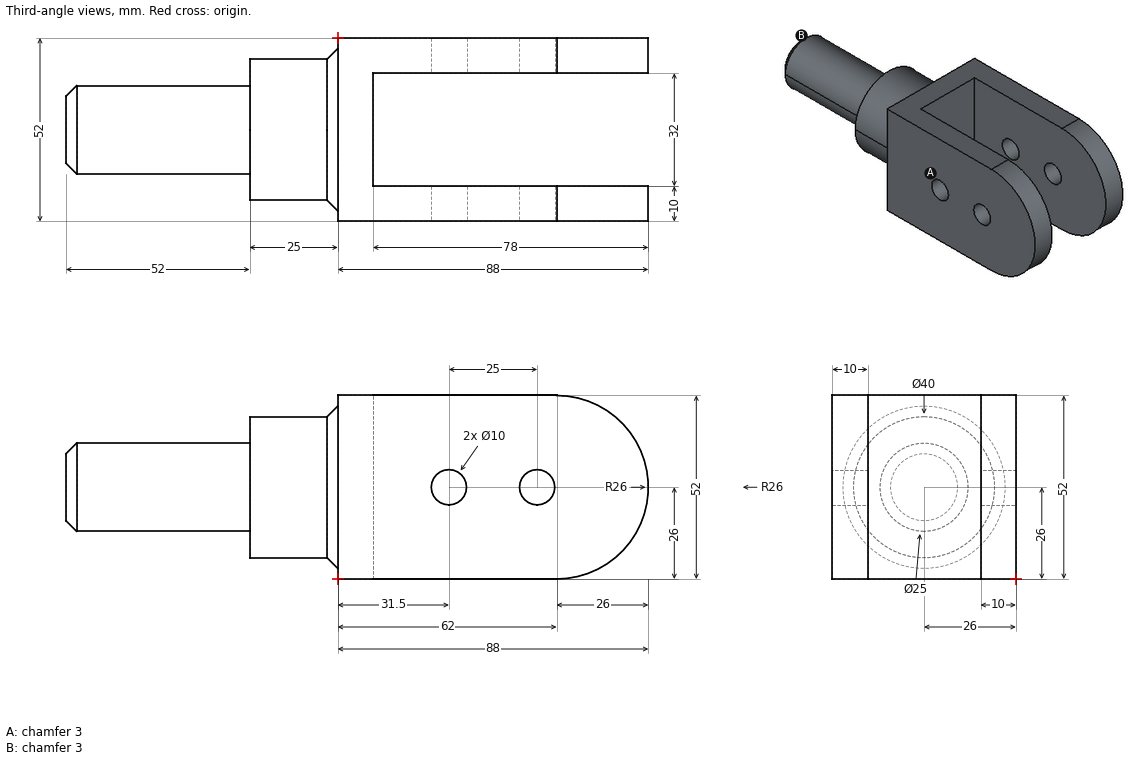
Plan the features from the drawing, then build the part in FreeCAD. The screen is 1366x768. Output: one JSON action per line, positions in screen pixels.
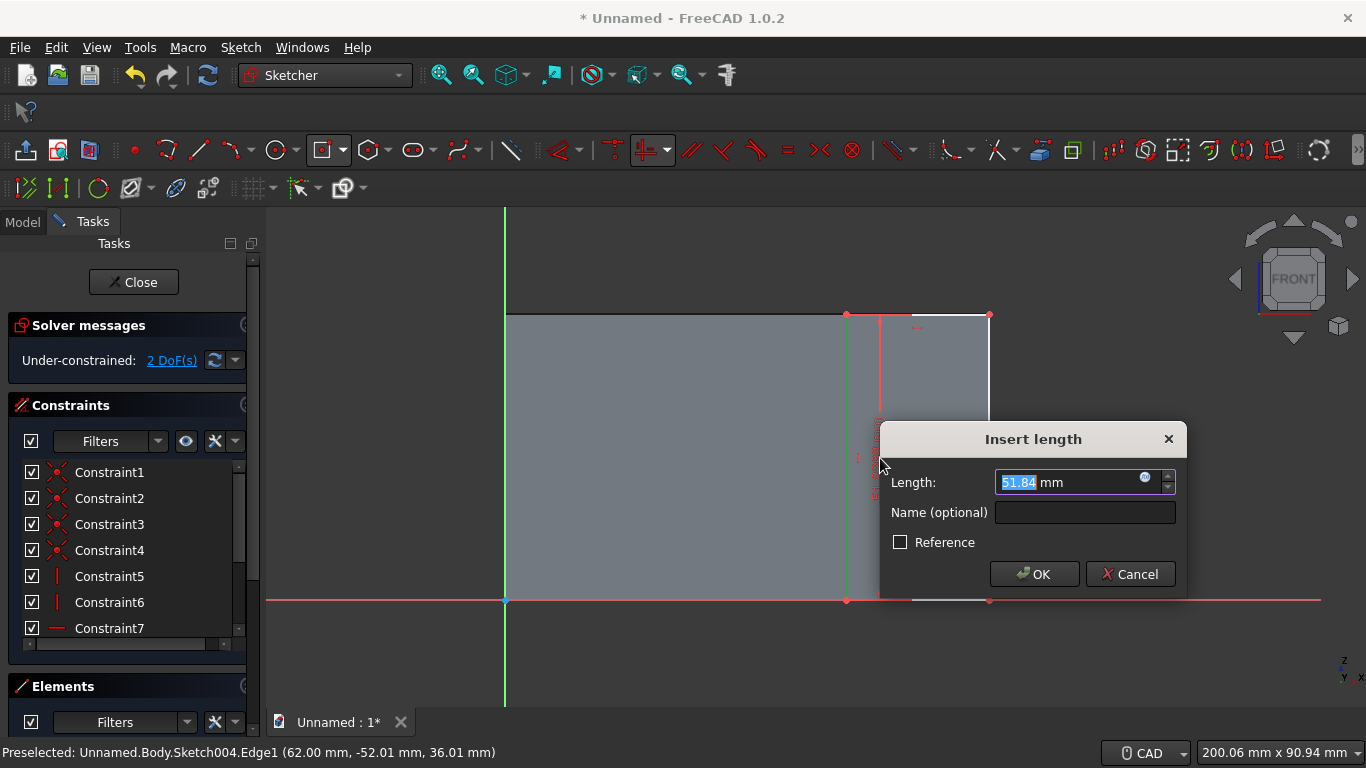
{"action": "type", "text": "52"}
{"action": "key", "text": "Return"}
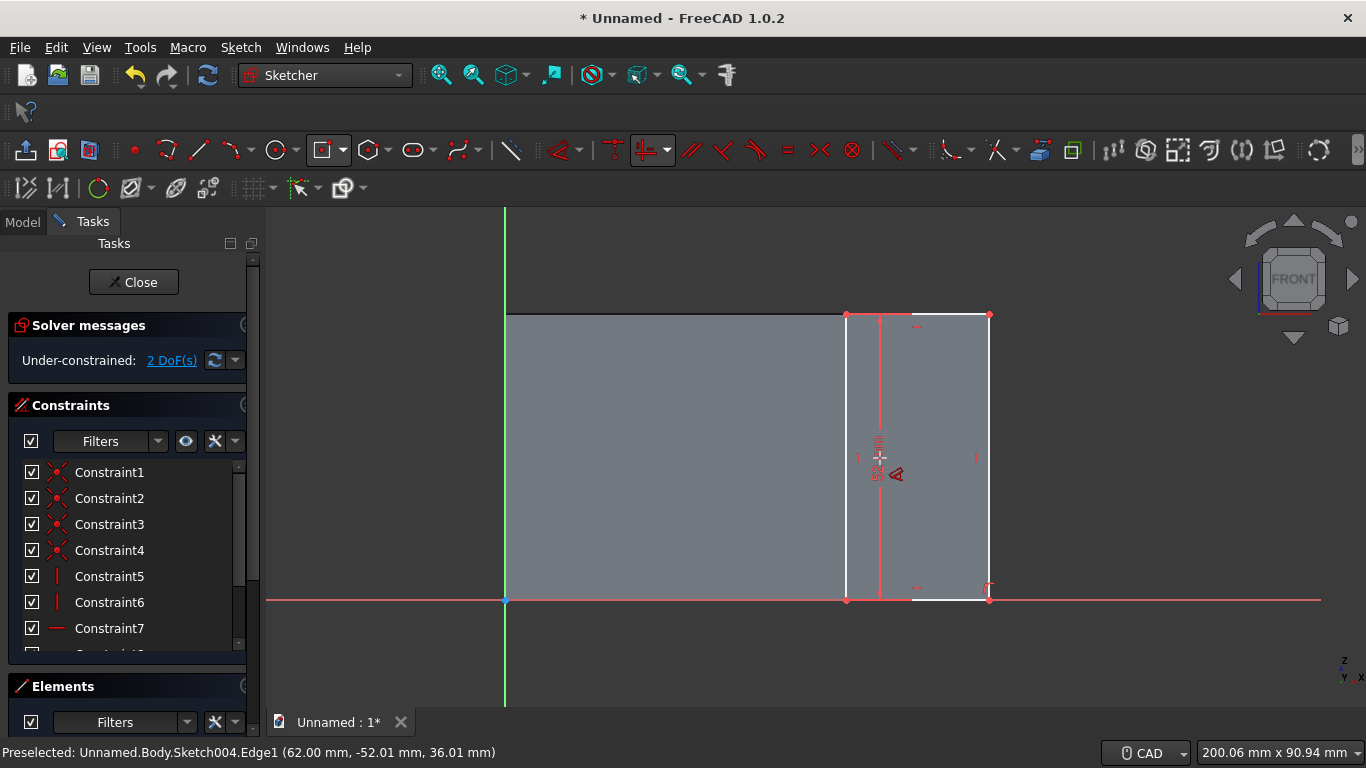
{"action": "left_click", "coordinate": [889, 600]}
{"action": "left_click", "coordinate": [917, 634]}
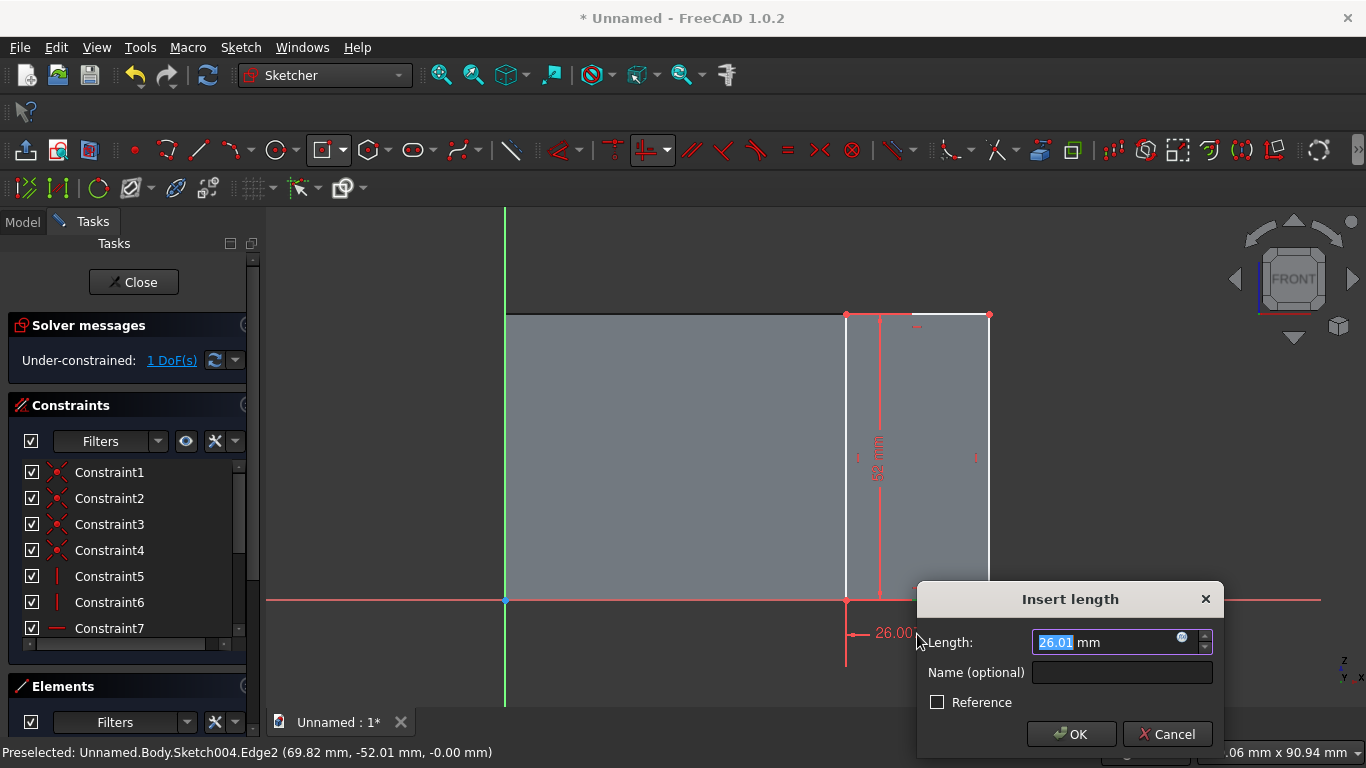
{"action": "type", "text": "26"}
{"action": "key", "text": "Return"}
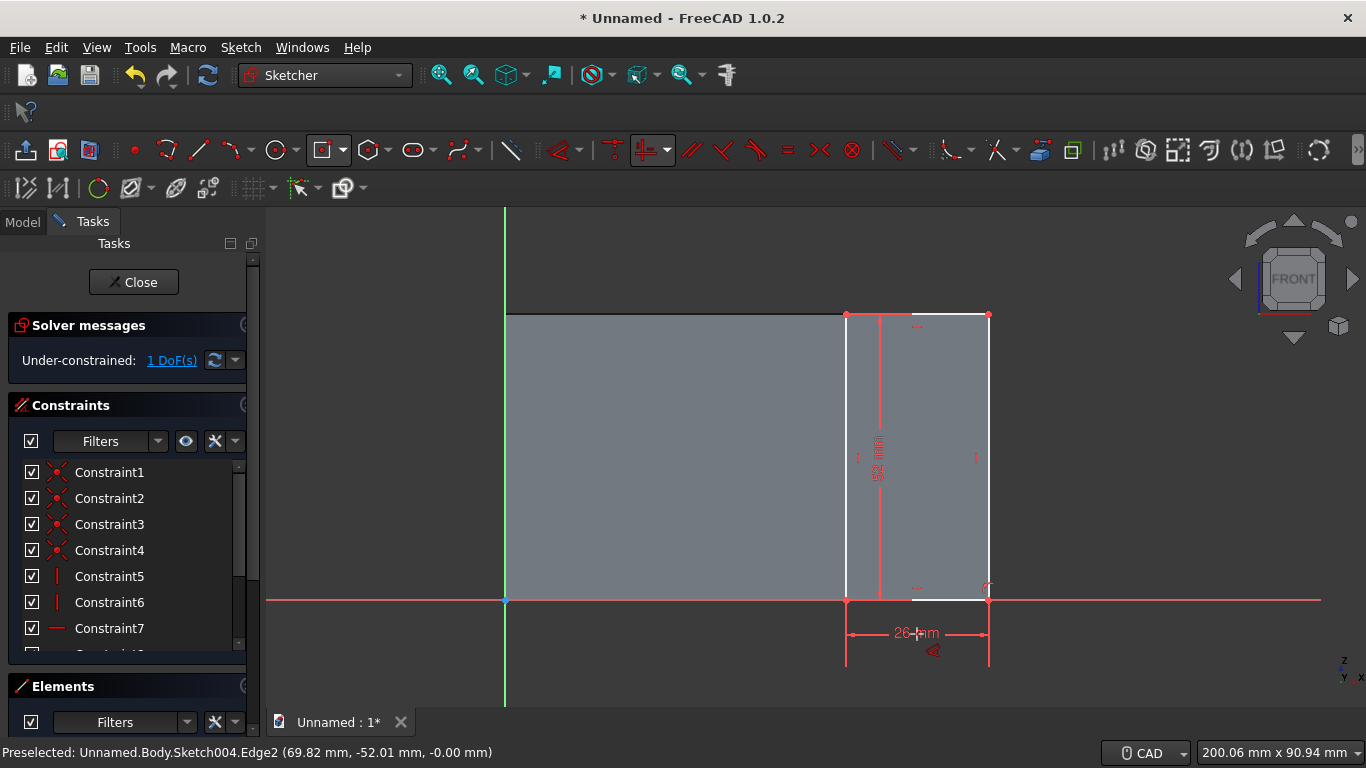
{"action": "left_click", "coordinate": [846, 314]}
{"action": "left_click", "coordinate": [676, 634]}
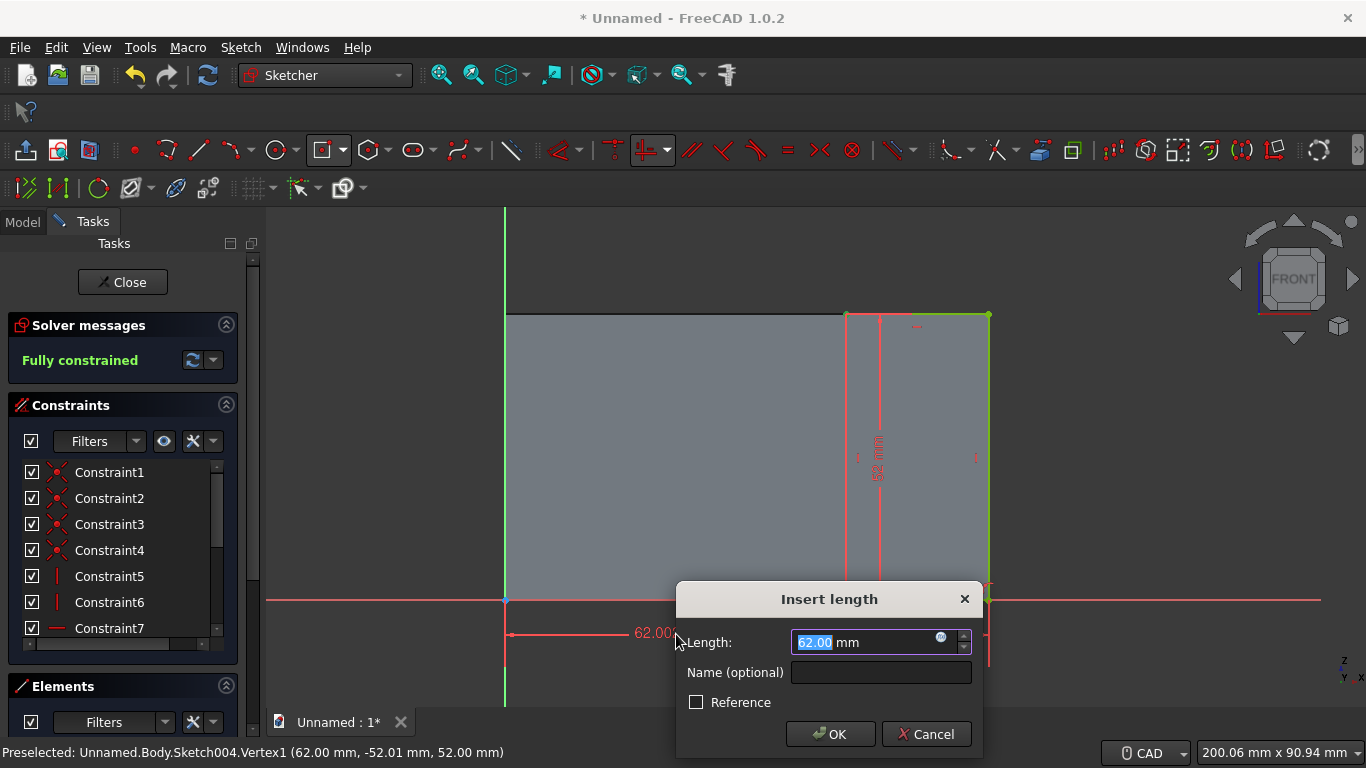
{"action": "type", "text": "62"}
{"action": "key", "text": "Return"}
{"action": "key", "text": "Escape"}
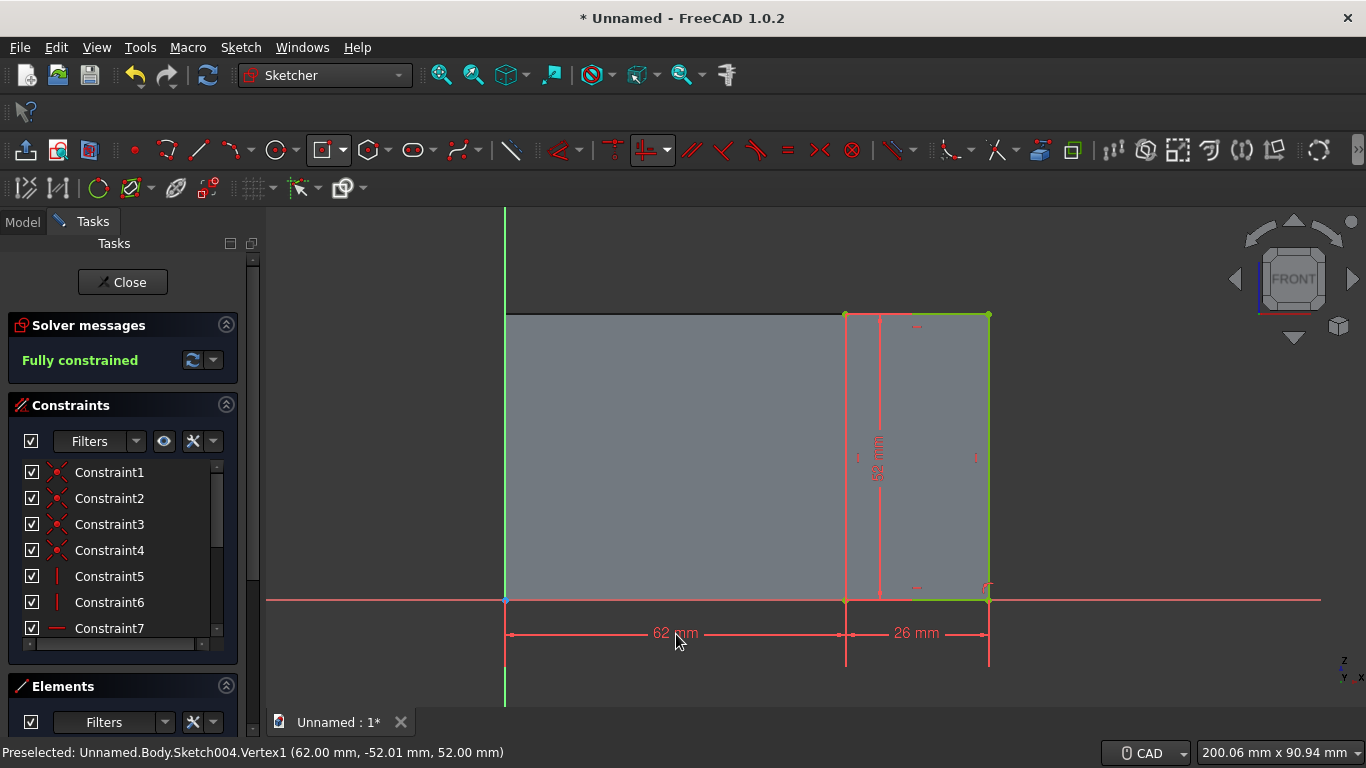
{"action": "left_click", "coordinate": [123, 282]}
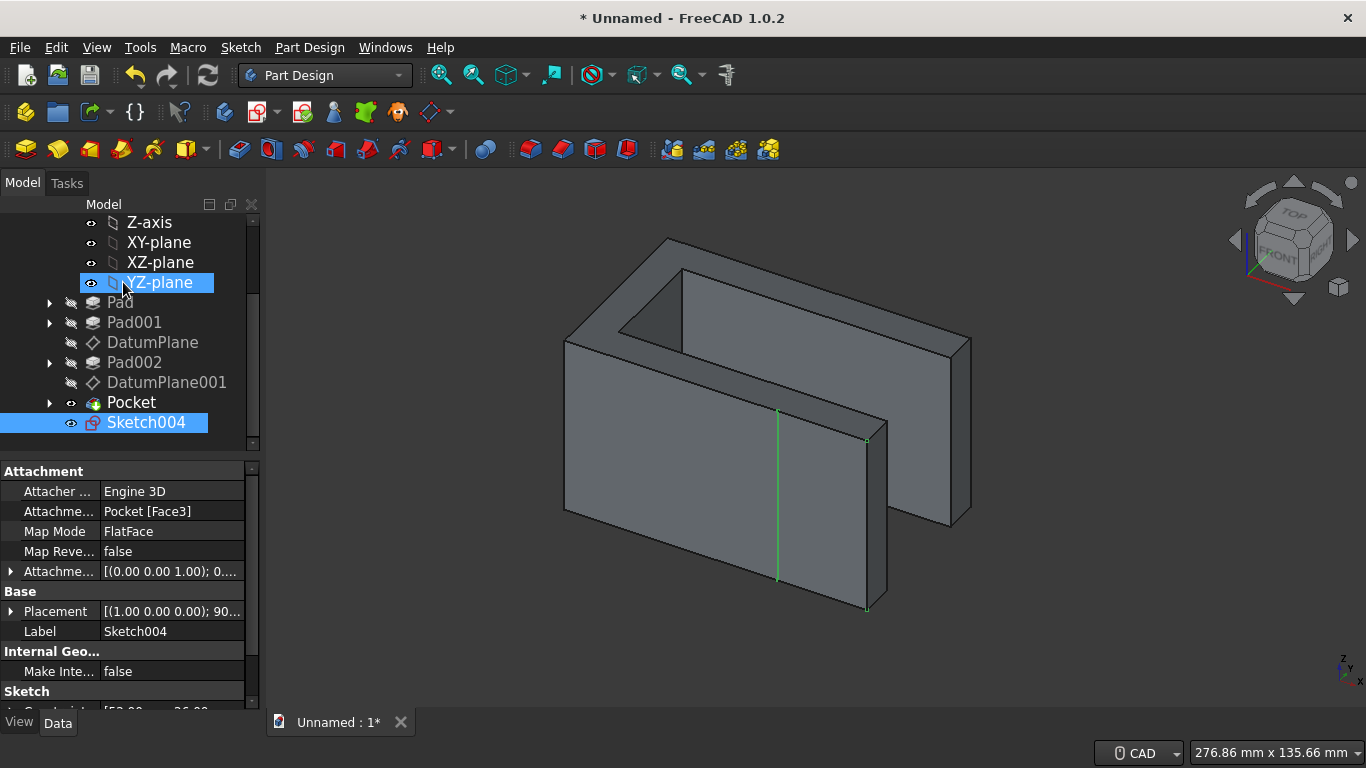
{"action": "left_click", "coordinate": [240, 150]}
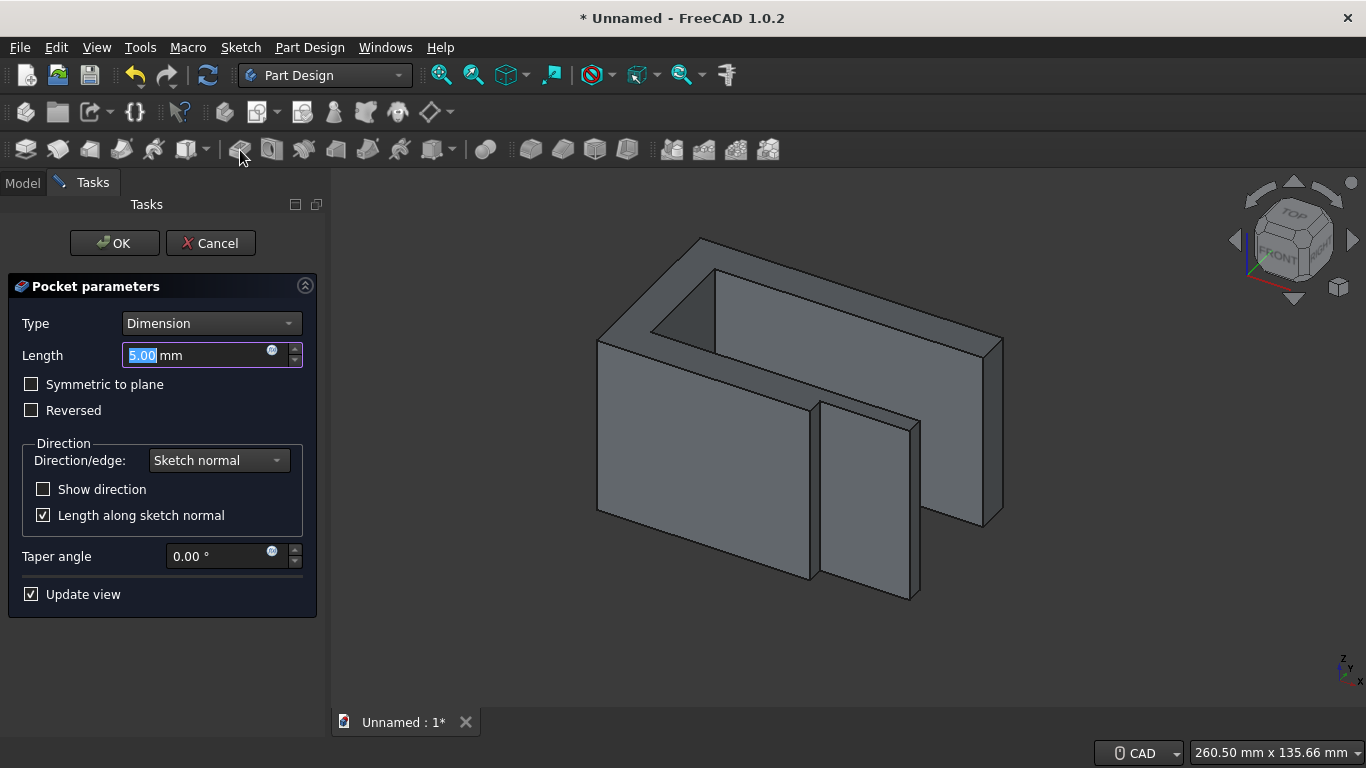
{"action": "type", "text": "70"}
{"action": "key", "text": "Tab"}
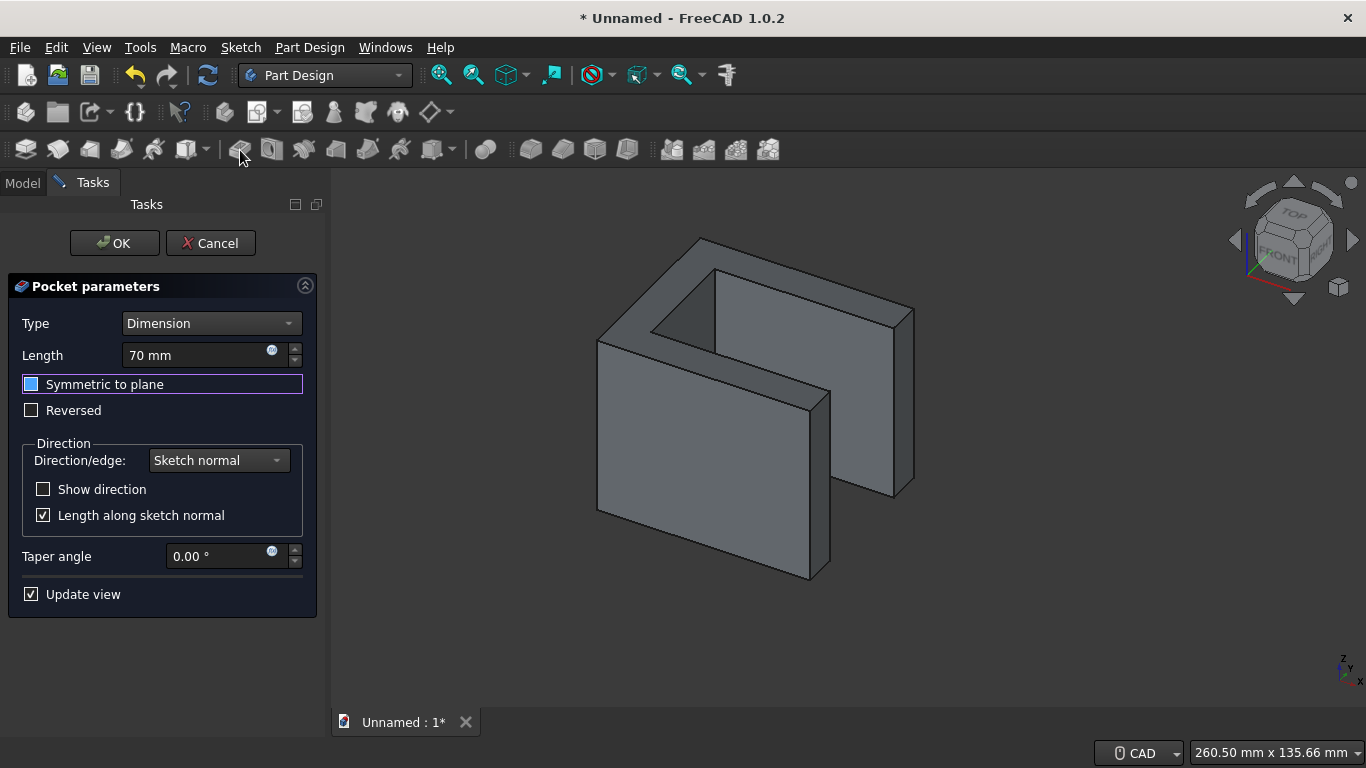
{"action": "left_click", "coordinate": [115, 243]}